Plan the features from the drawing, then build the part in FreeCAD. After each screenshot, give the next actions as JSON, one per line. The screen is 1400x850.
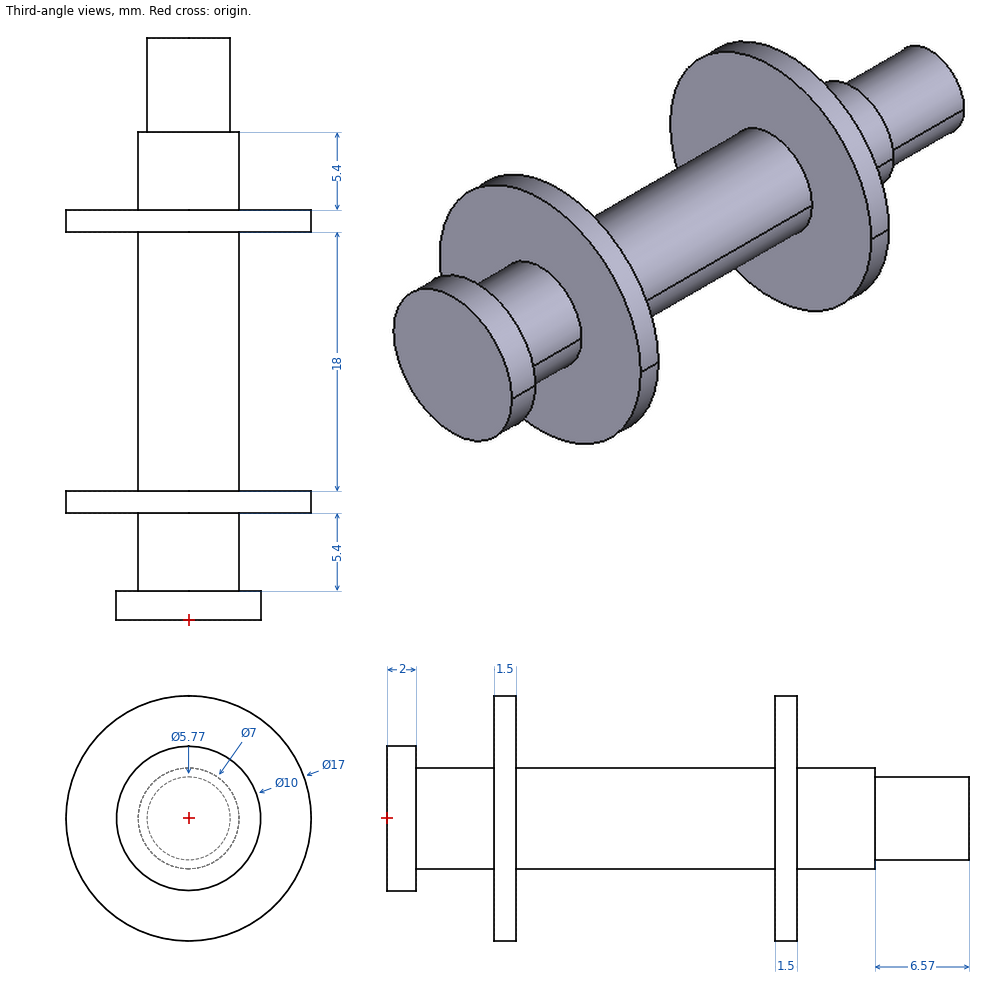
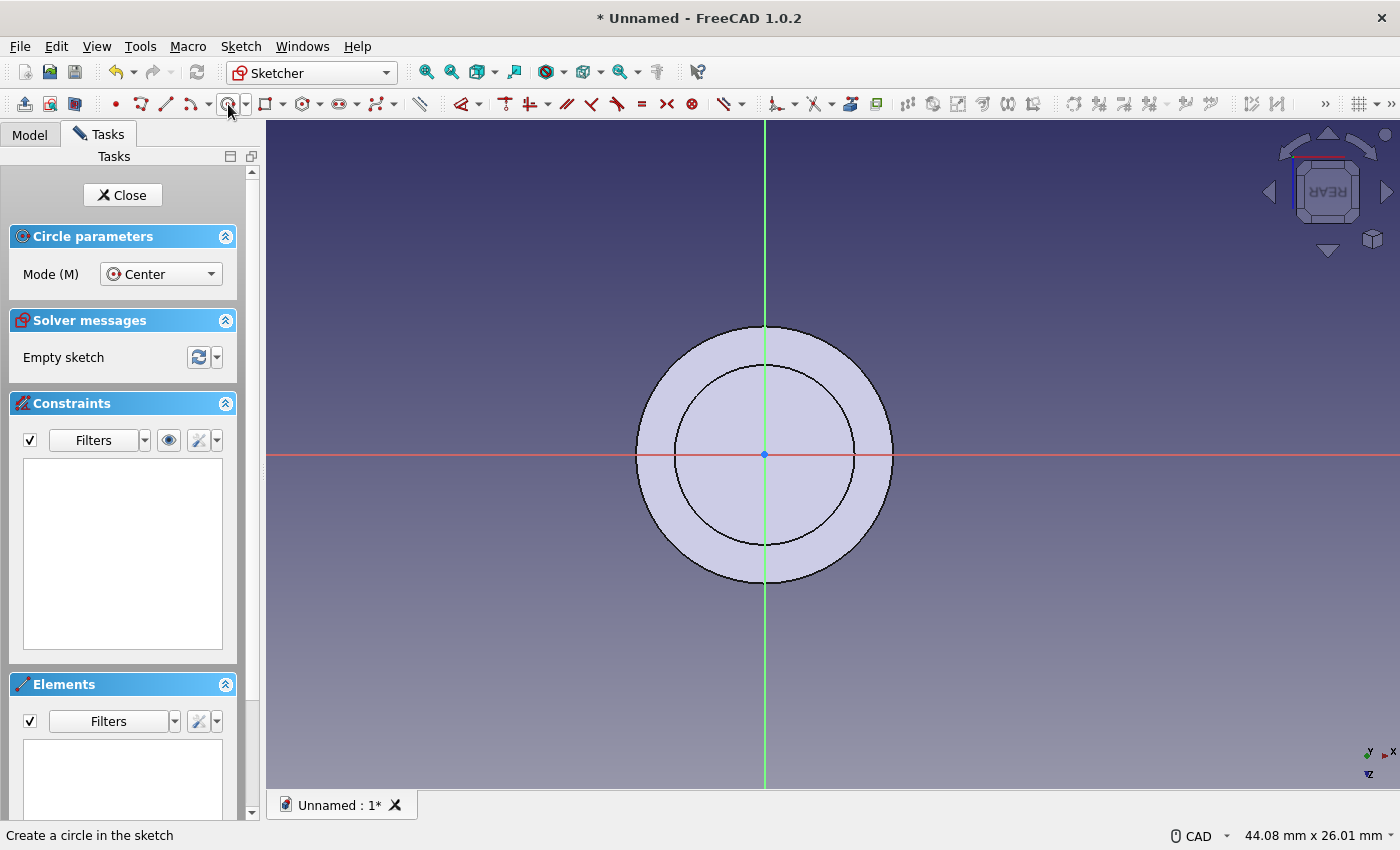
{"action": "left_click", "coordinate": [765, 455]}
{"action": "left_click", "coordinate": [919, 300]}
{"action": "key", "text": "Escape"}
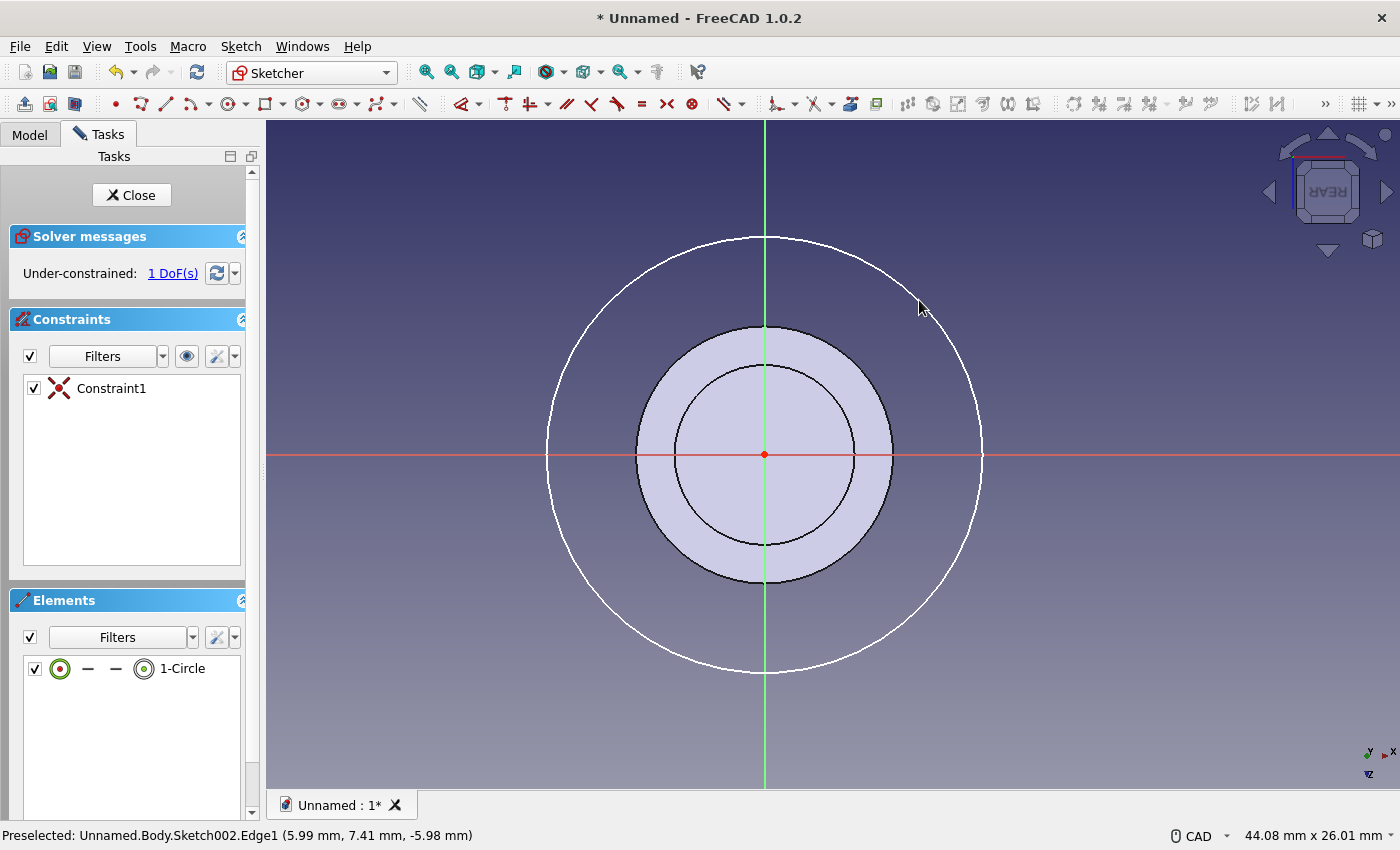
{"action": "left_click", "coordinate": [460, 104]}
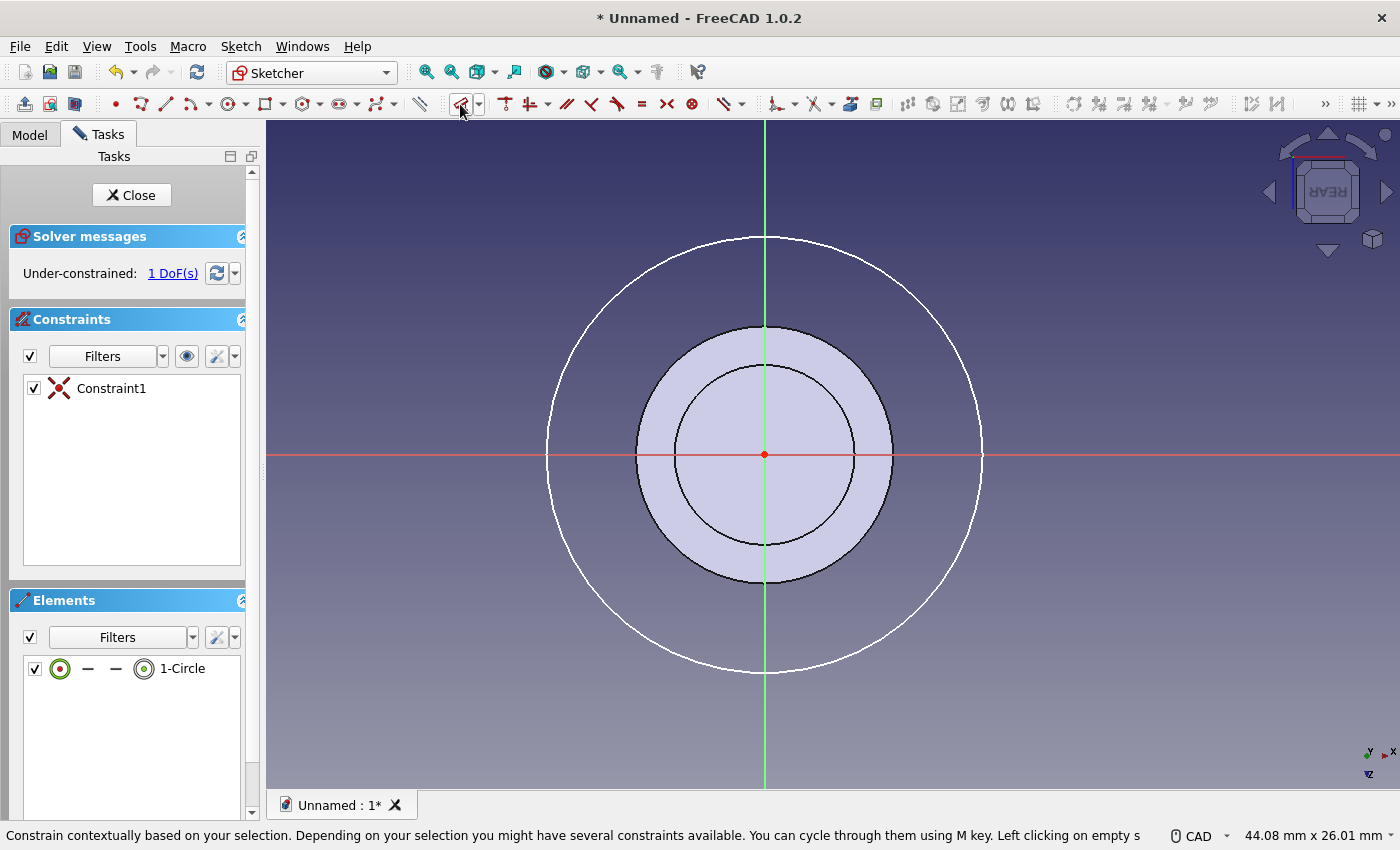
{"action": "left_click", "coordinate": [918, 300]}
{"action": "left_click", "coordinate": [941, 277]}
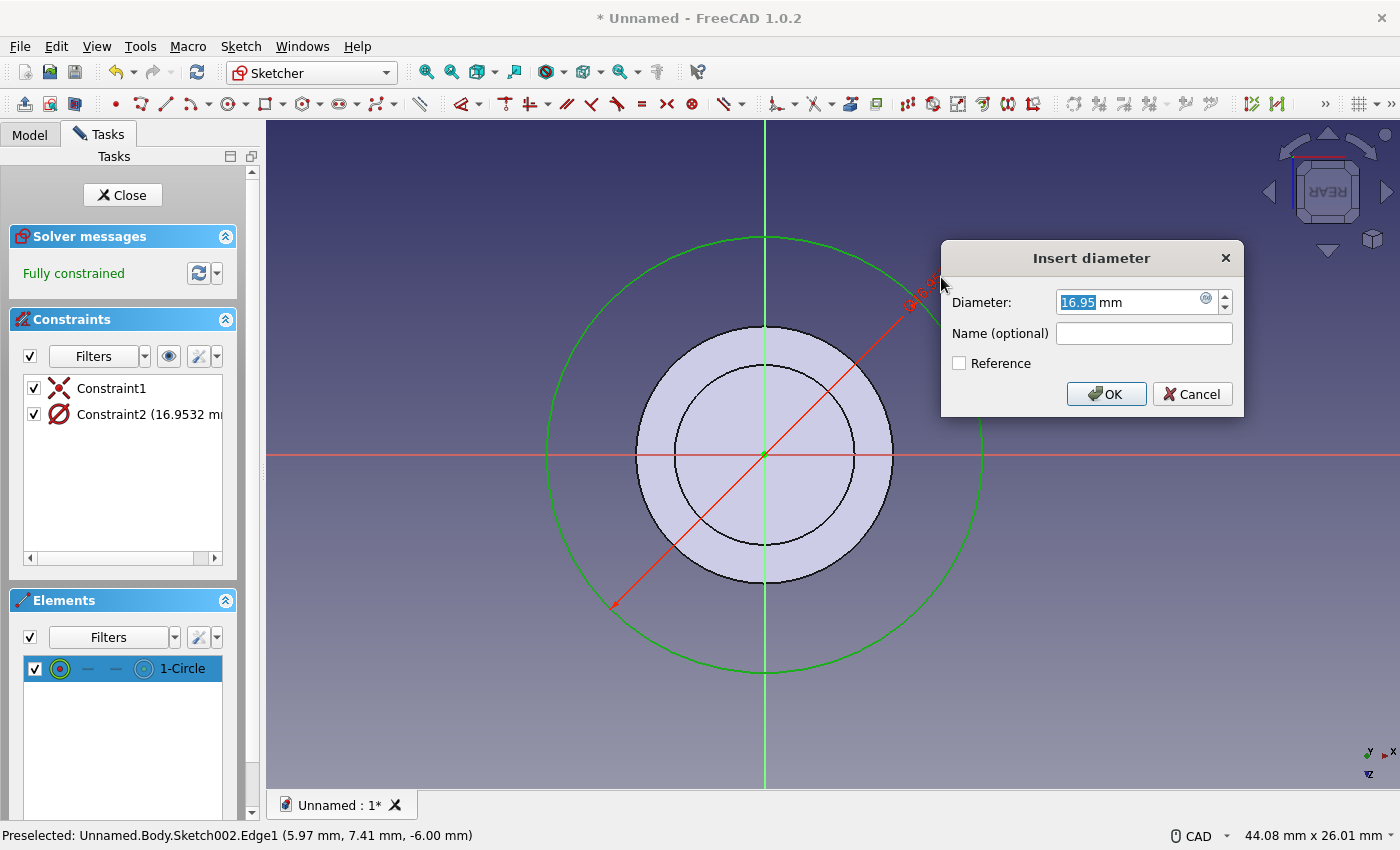
{"action": "type", "text": "17"}
{"action": "key", "text": "Return"}
{"action": "key", "text": "Escape"}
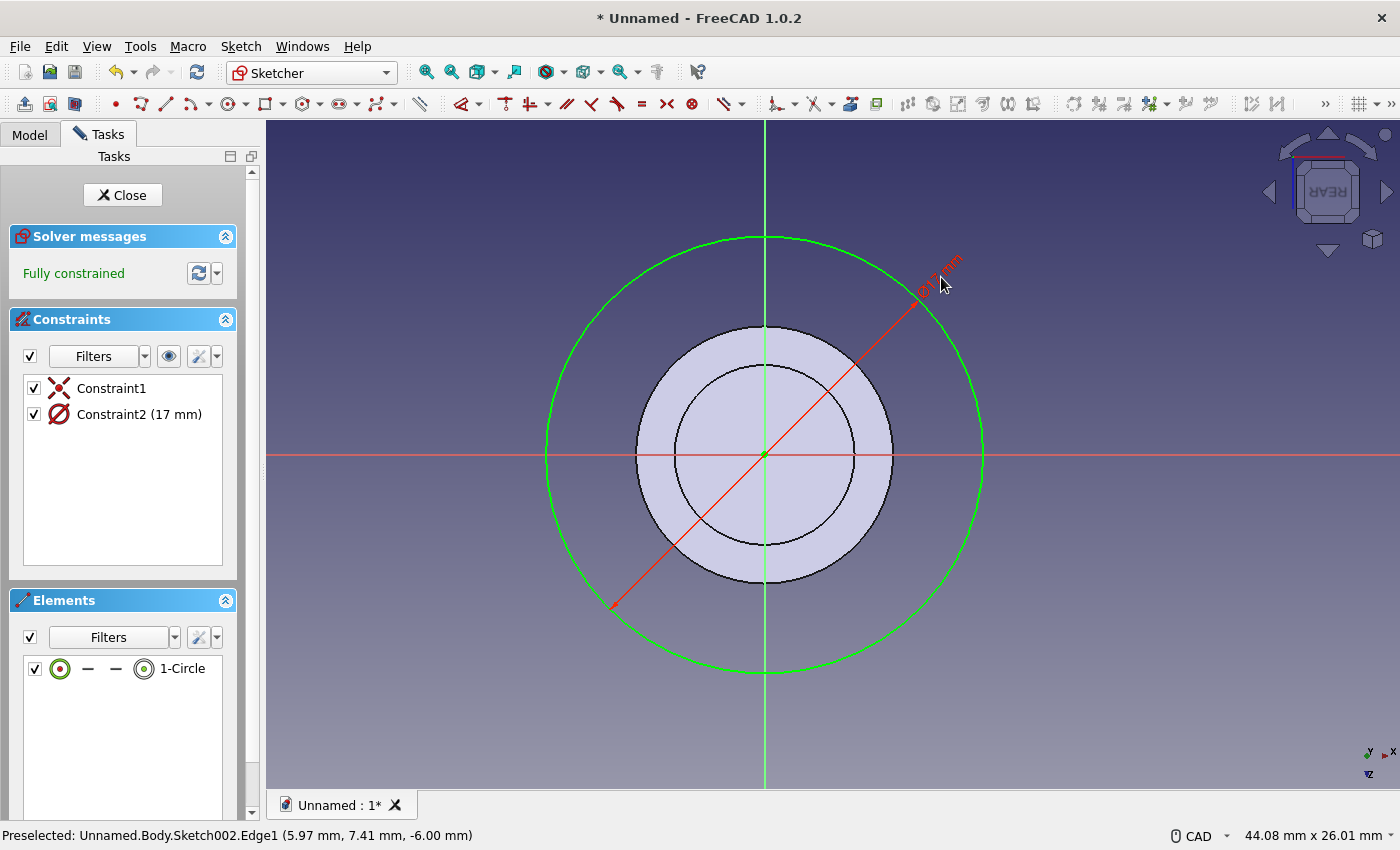
{"action": "left_click", "coordinate": [123, 195]}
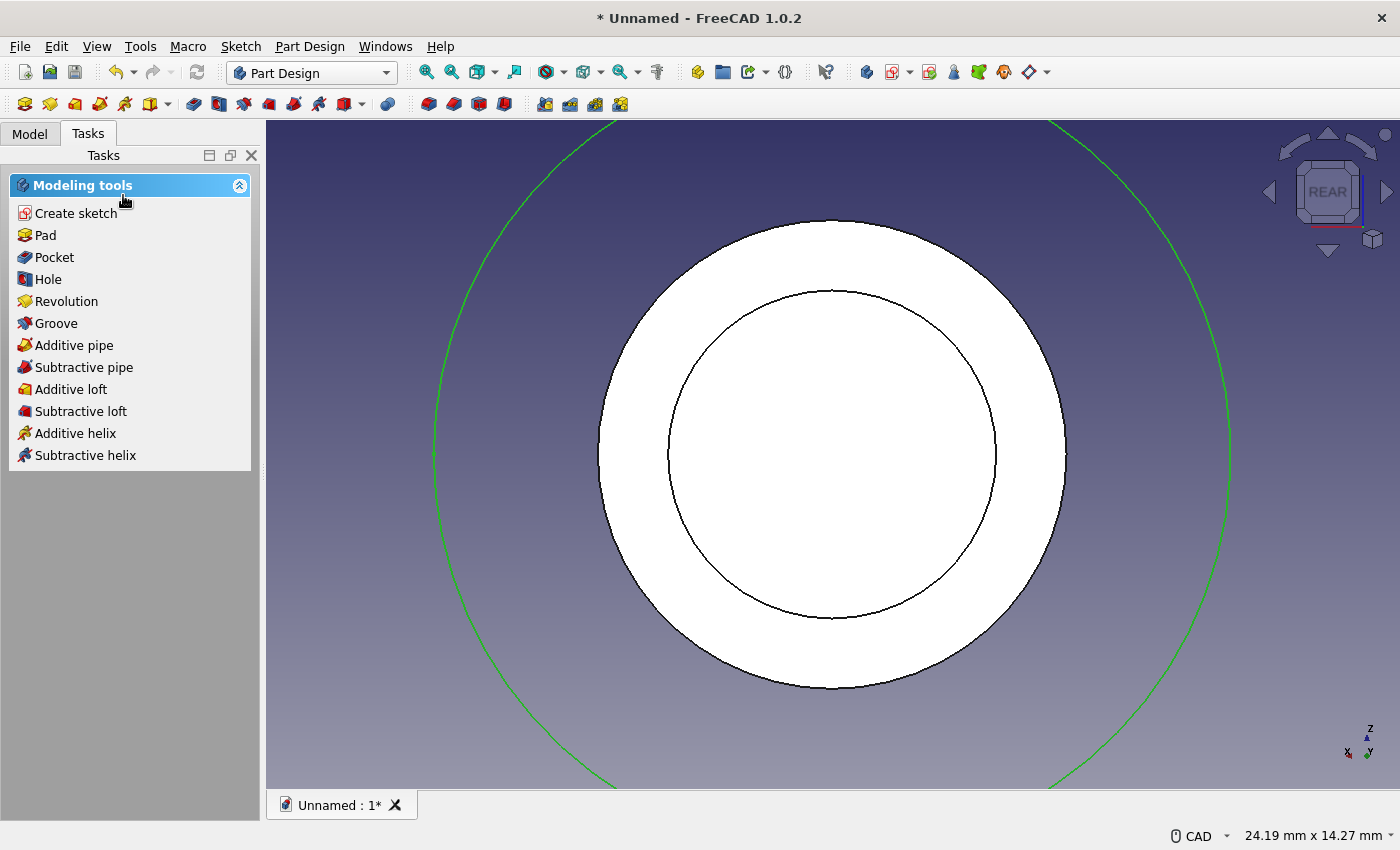
{"action": "left_click", "coordinate": [25, 104]}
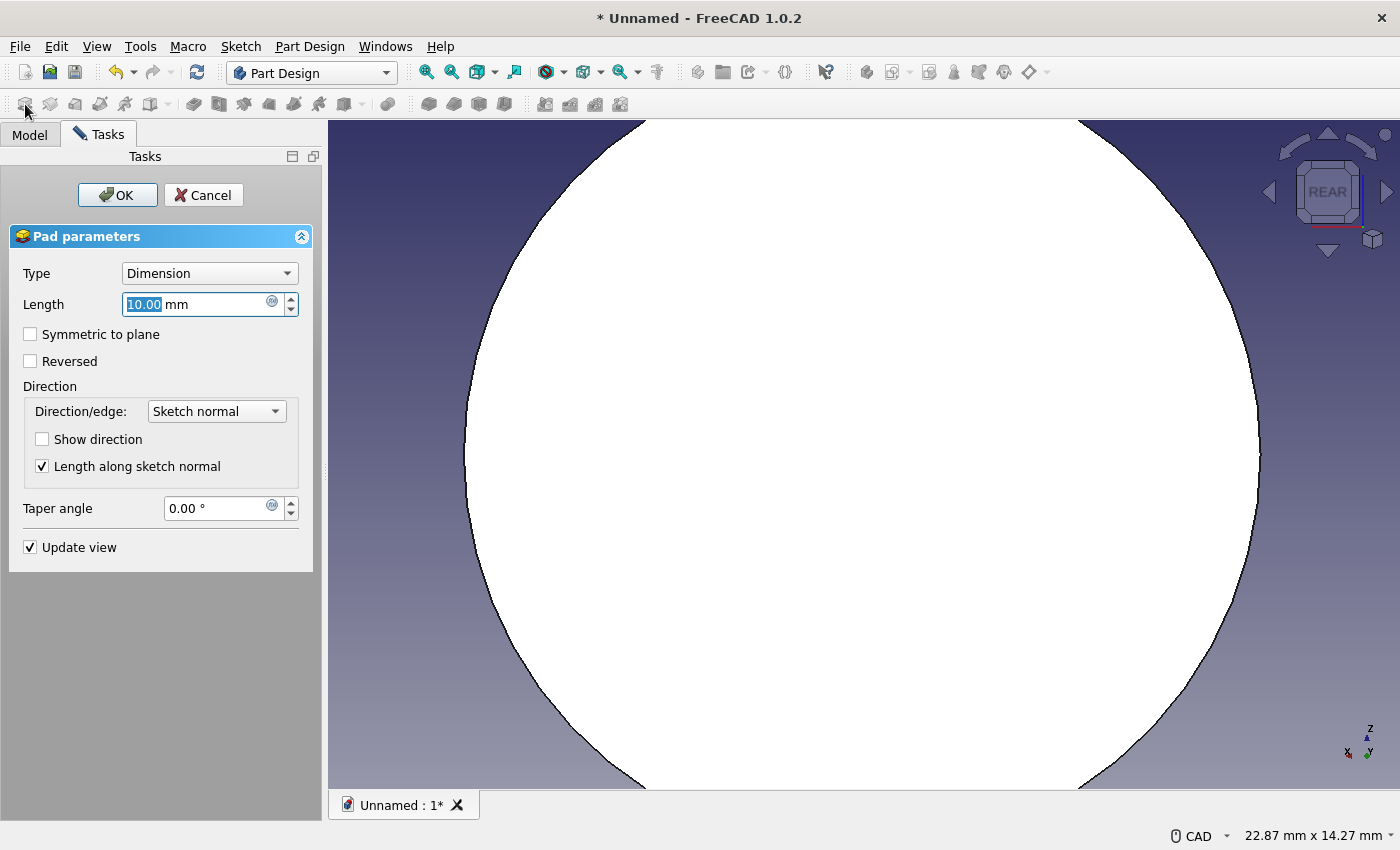
{"action": "type", "text": "1.5"}
{"action": "key", "text": "Tab"}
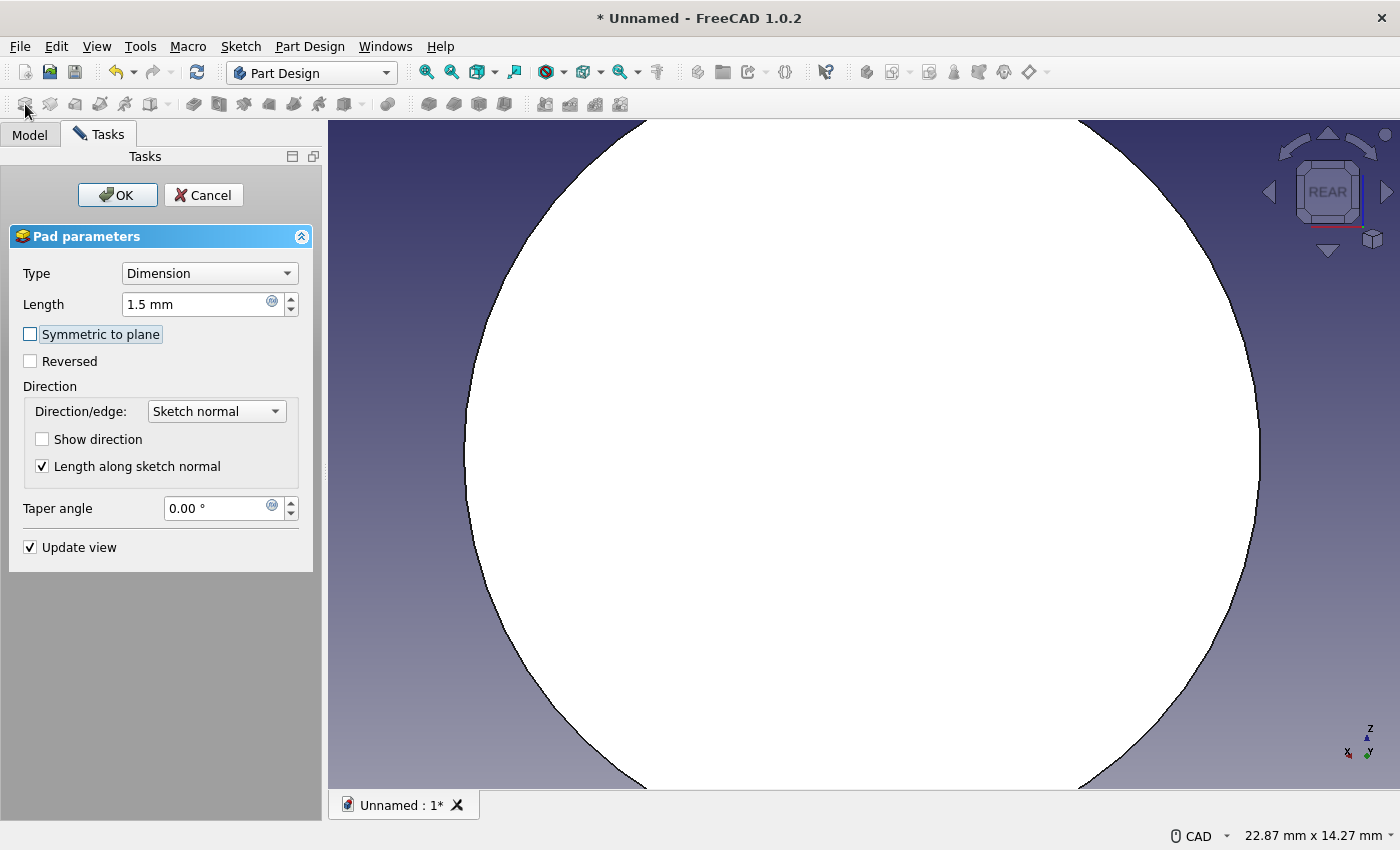
{"action": "left_click", "coordinate": [118, 195]}